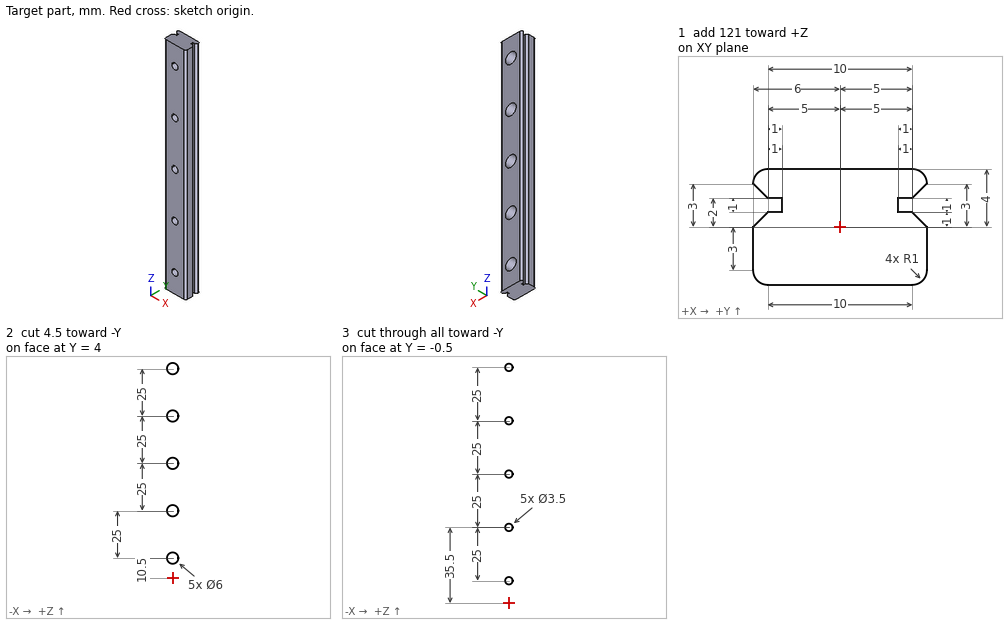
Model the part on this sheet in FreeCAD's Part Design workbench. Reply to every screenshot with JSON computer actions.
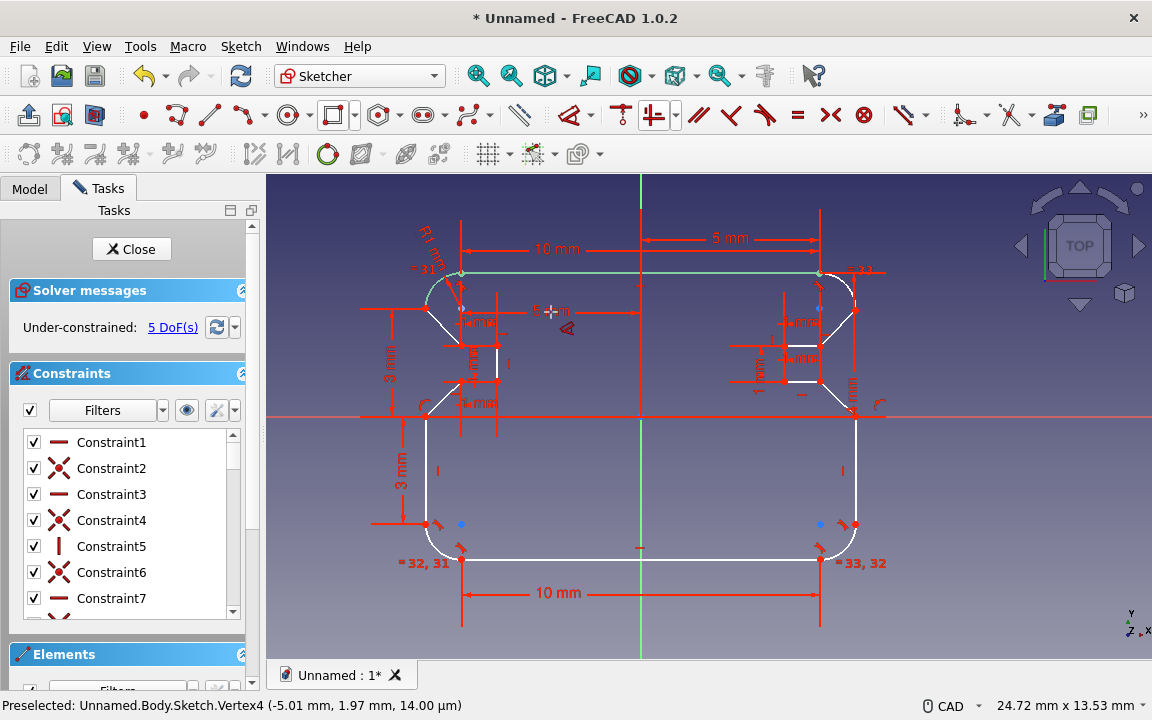
{"action": "left_click", "coordinate": [461, 346]}
{"action": "left_click", "coordinate": [675, 381]}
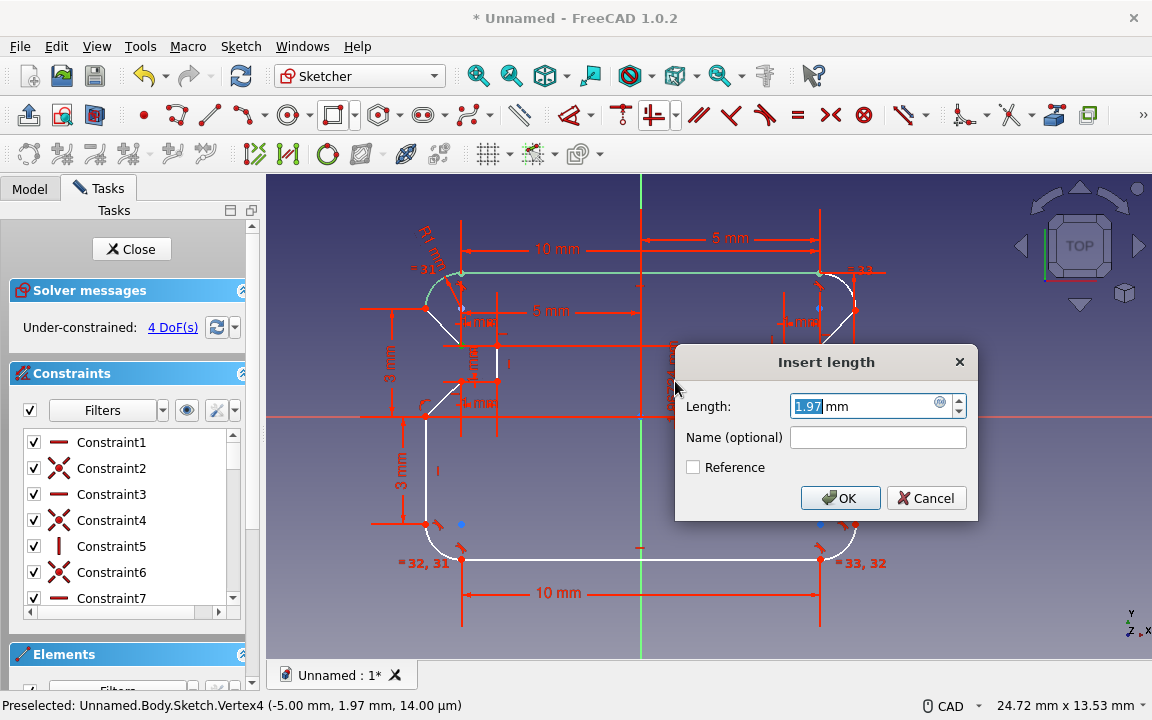
{"action": "type", "text": "2"}
{"action": "key", "text": "Return"}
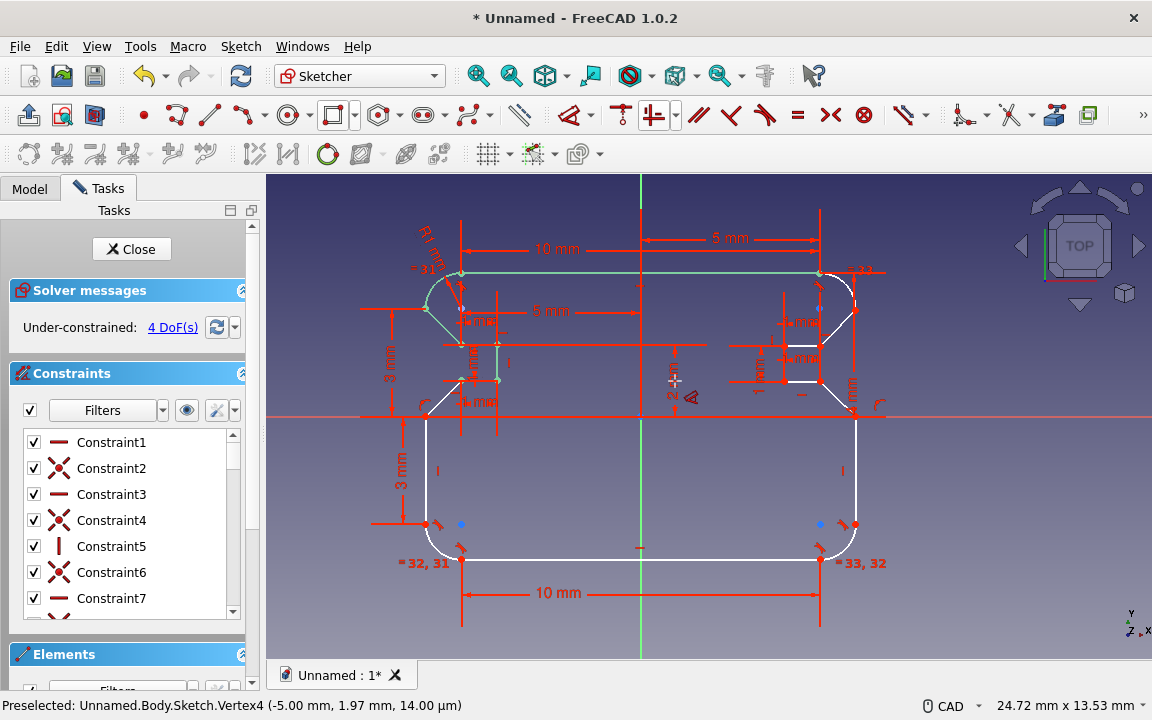
{"action": "left_click", "coordinate": [426, 416]}
{"action": "left_click", "coordinate": [533, 450]}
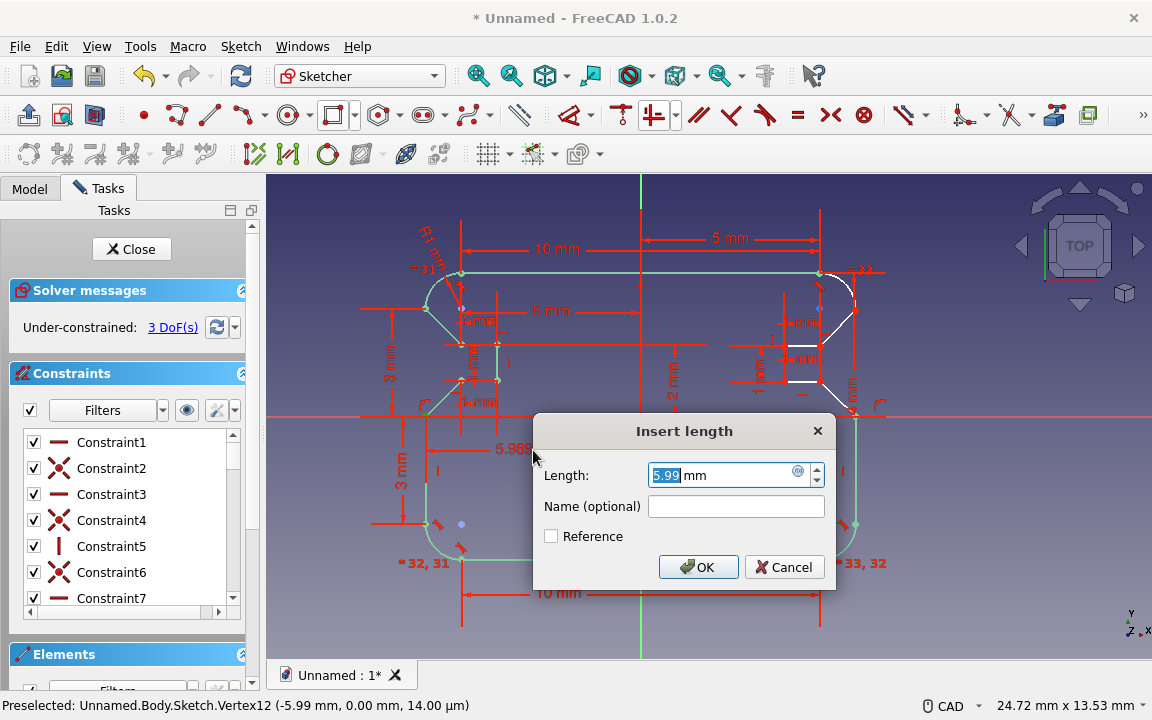
{"action": "type", "text": "6"}
{"action": "key", "text": "Return"}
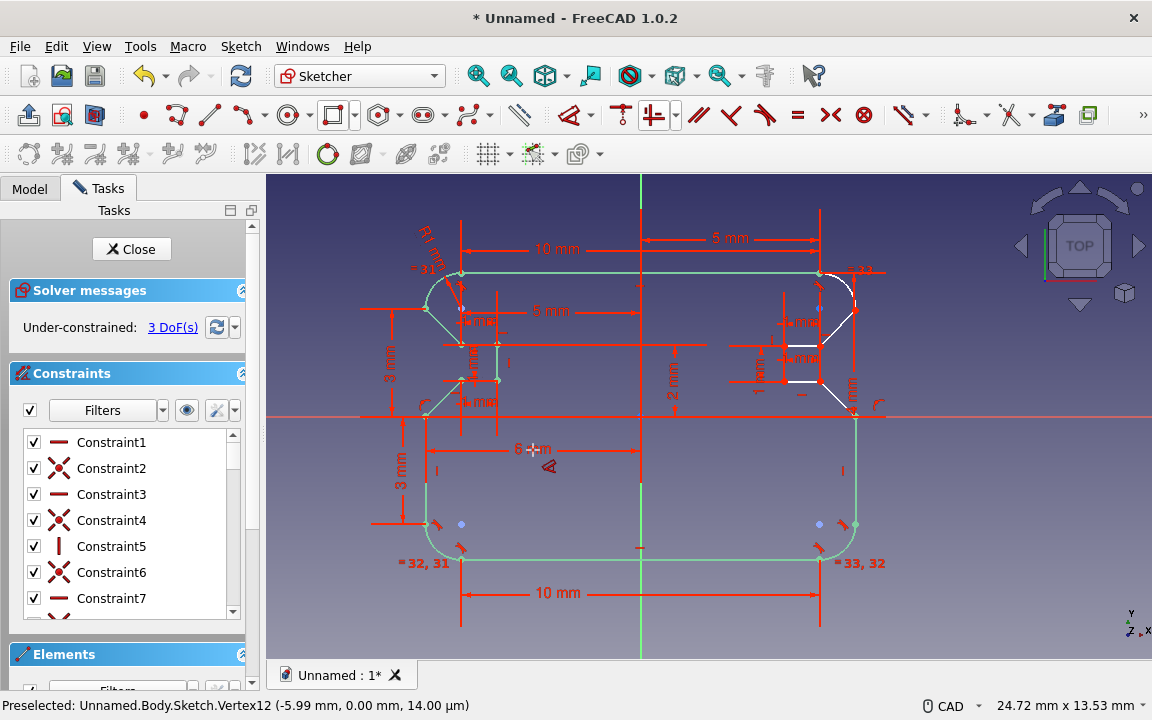
{"action": "left_click", "coordinate": [820, 382]}
{"action": "left_click", "coordinate": [730, 348]}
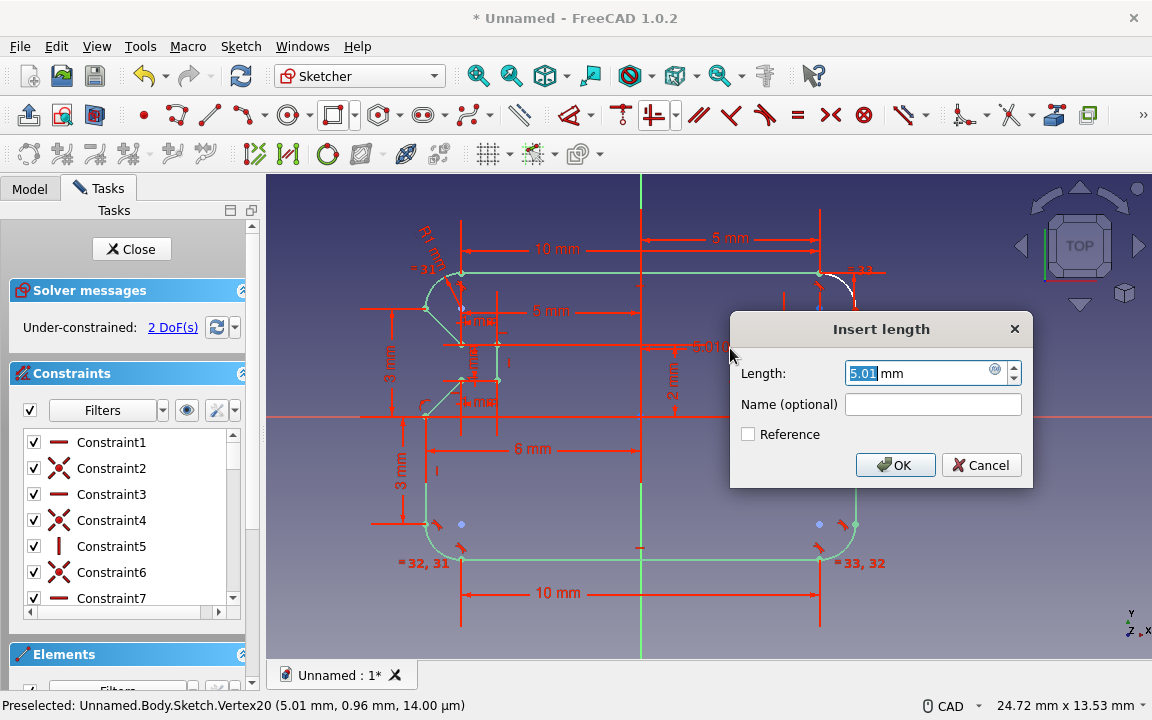
{"action": "type", "text": "5"}
{"action": "key", "text": "Return"}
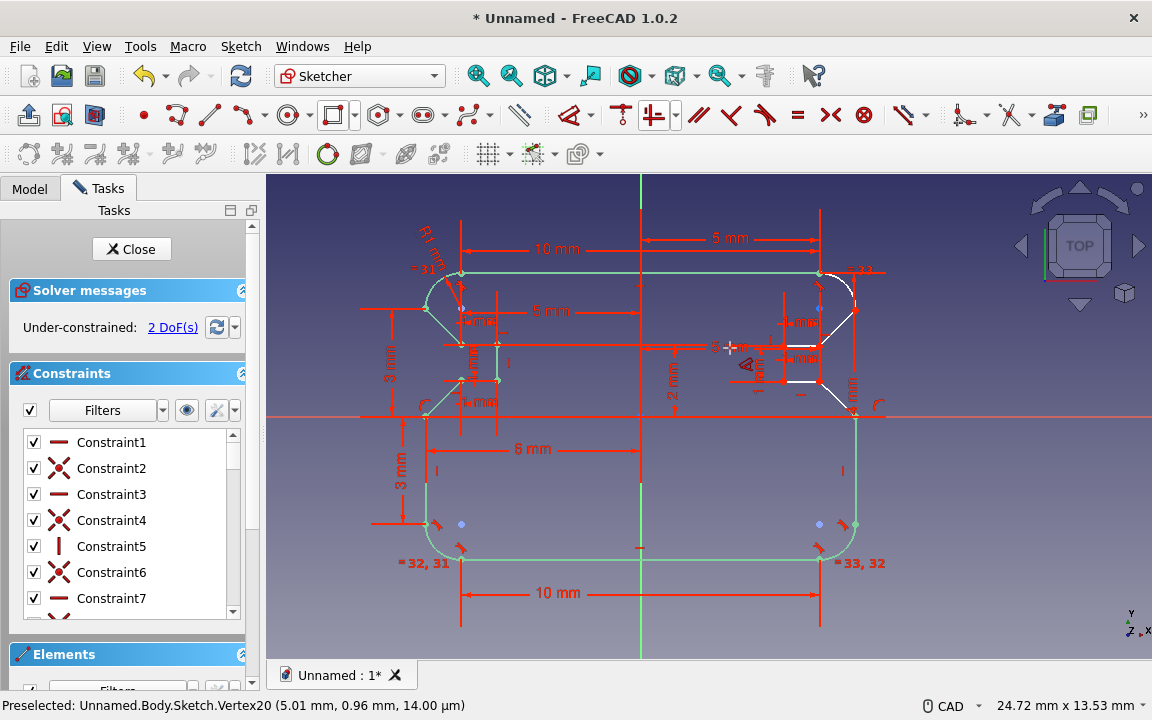
{"action": "left_click", "coordinate": [820, 382]}
{"action": "left_click", "coordinate": [583, 399]}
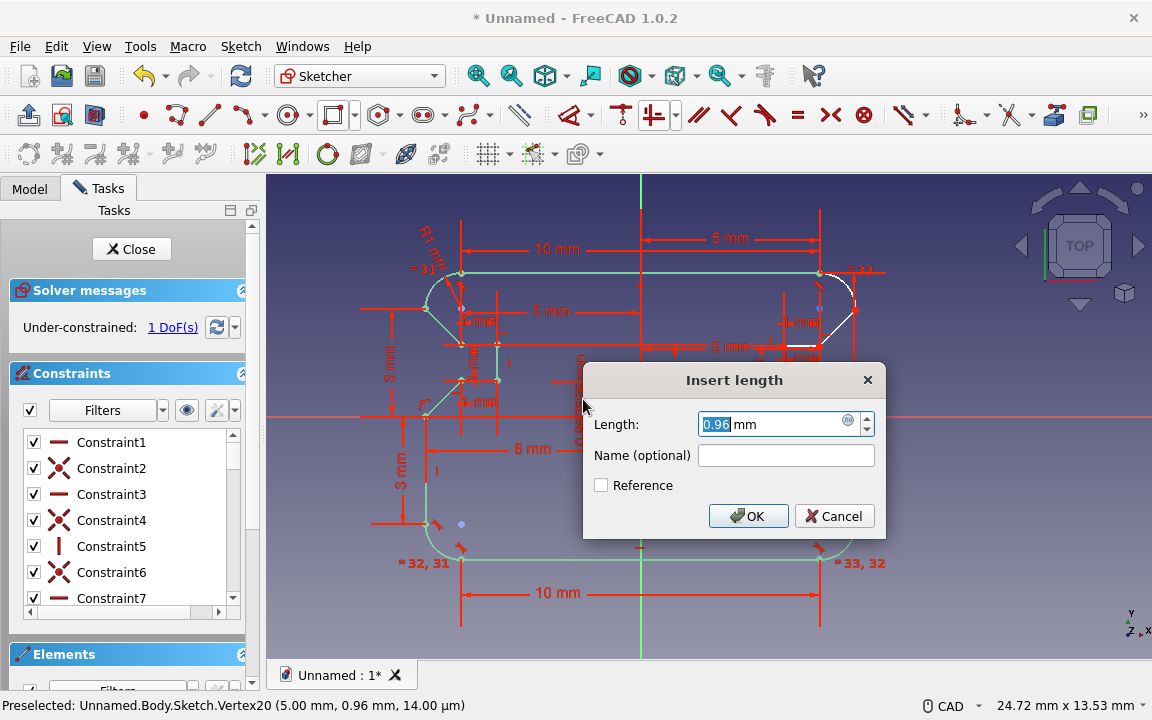
{"action": "type", "text": "1"}
{"action": "key", "text": "Return"}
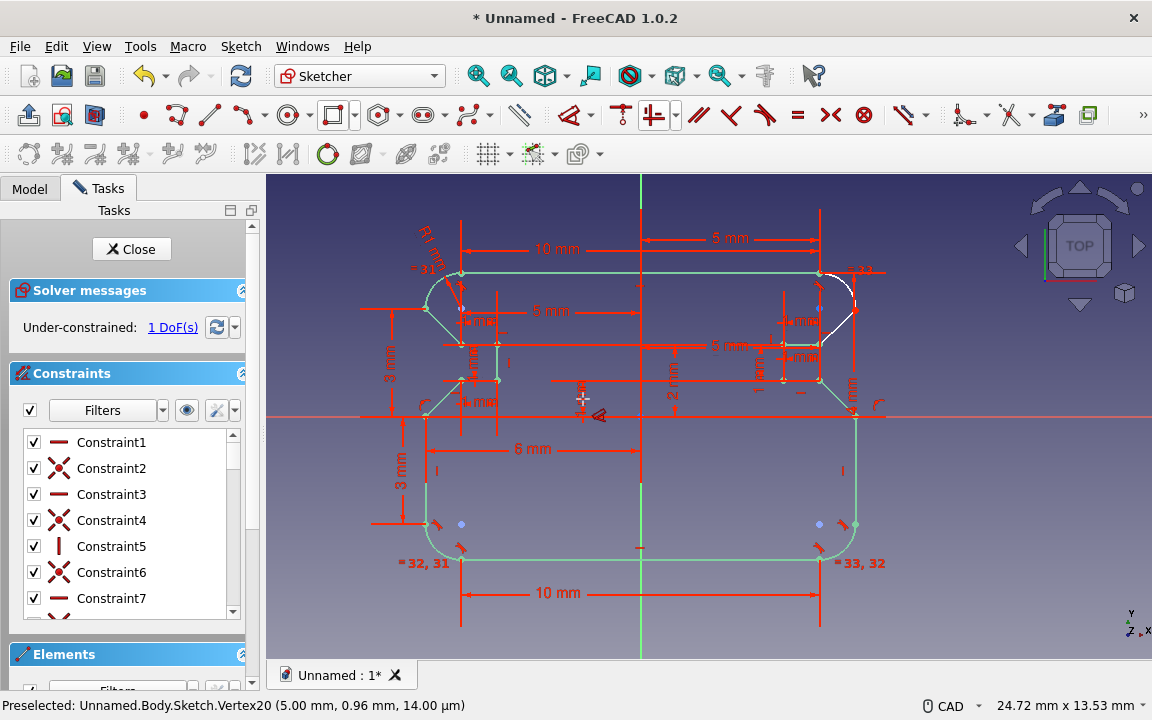
{"action": "left_click", "coordinate": [856, 310]}
{"action": "left_click", "coordinate": [890, 363]}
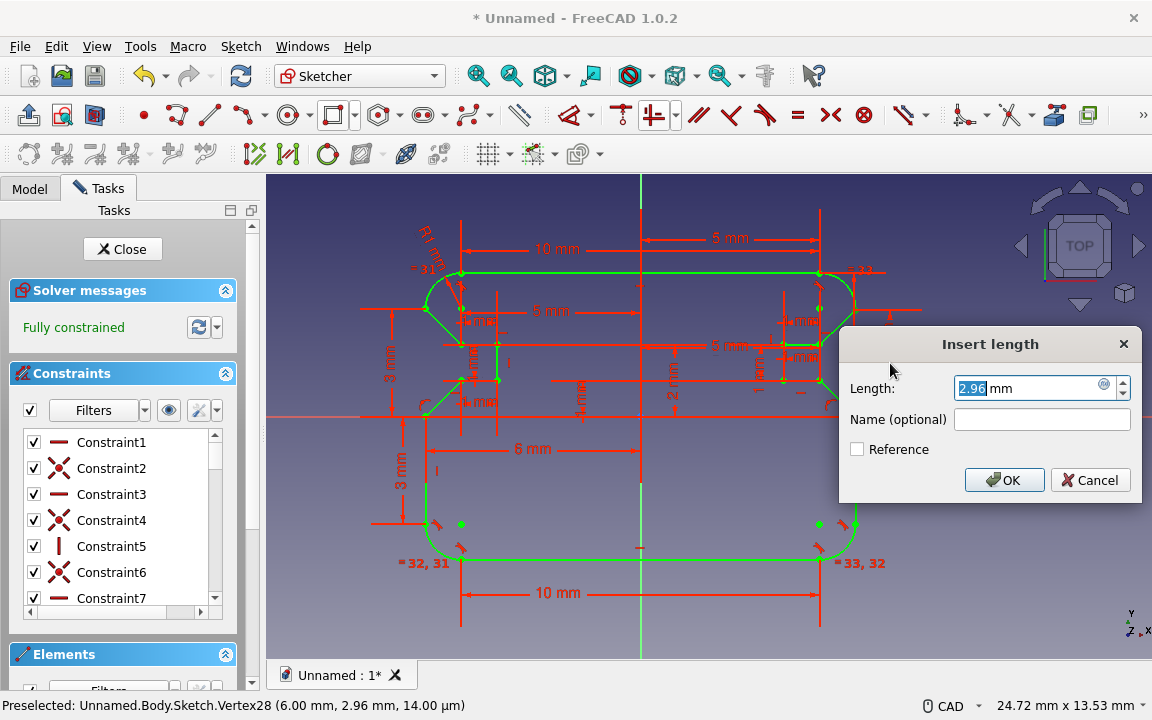
{"action": "type", "text": "3"}
{"action": "key", "text": "Return"}
{"action": "key", "text": "Escape"}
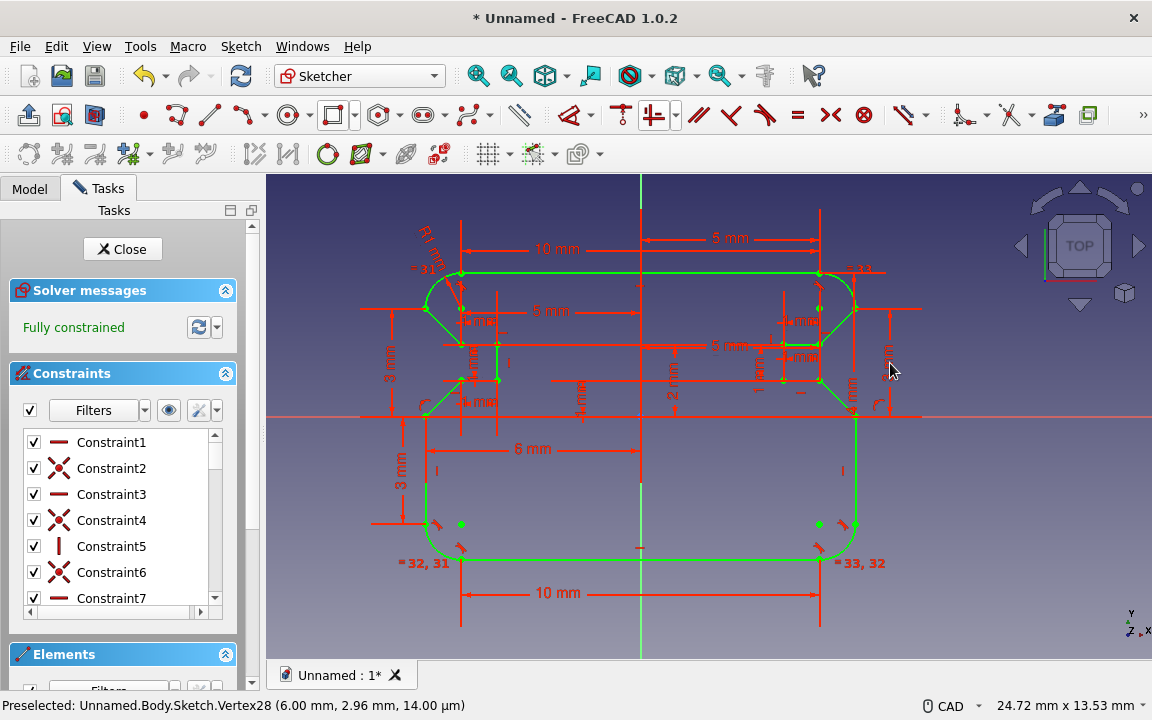
{"action": "left_click", "coordinate": [123, 249]}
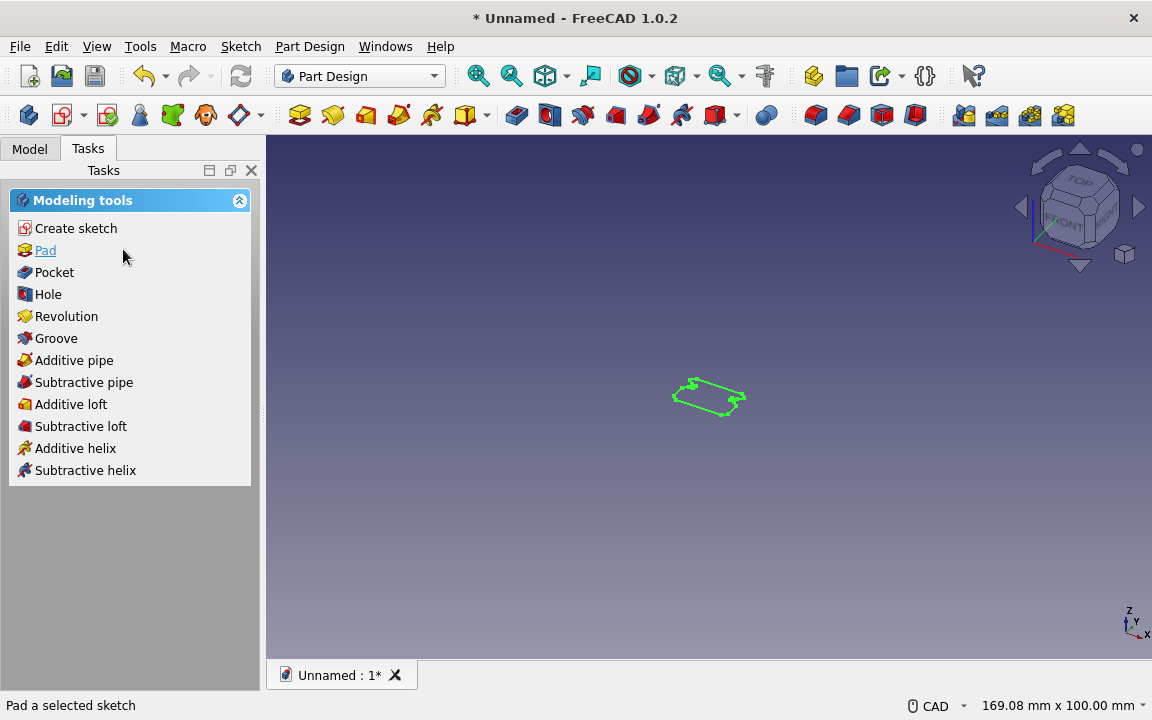
{"action": "left_click", "coordinate": [300, 116]}